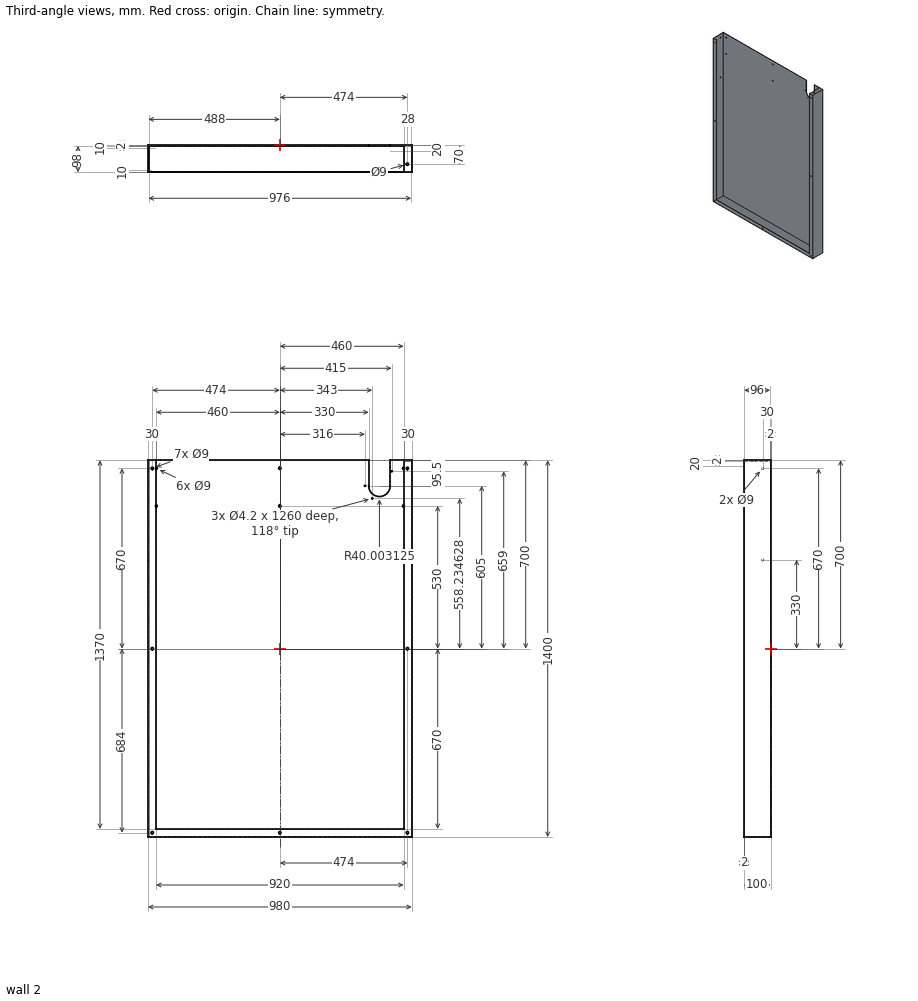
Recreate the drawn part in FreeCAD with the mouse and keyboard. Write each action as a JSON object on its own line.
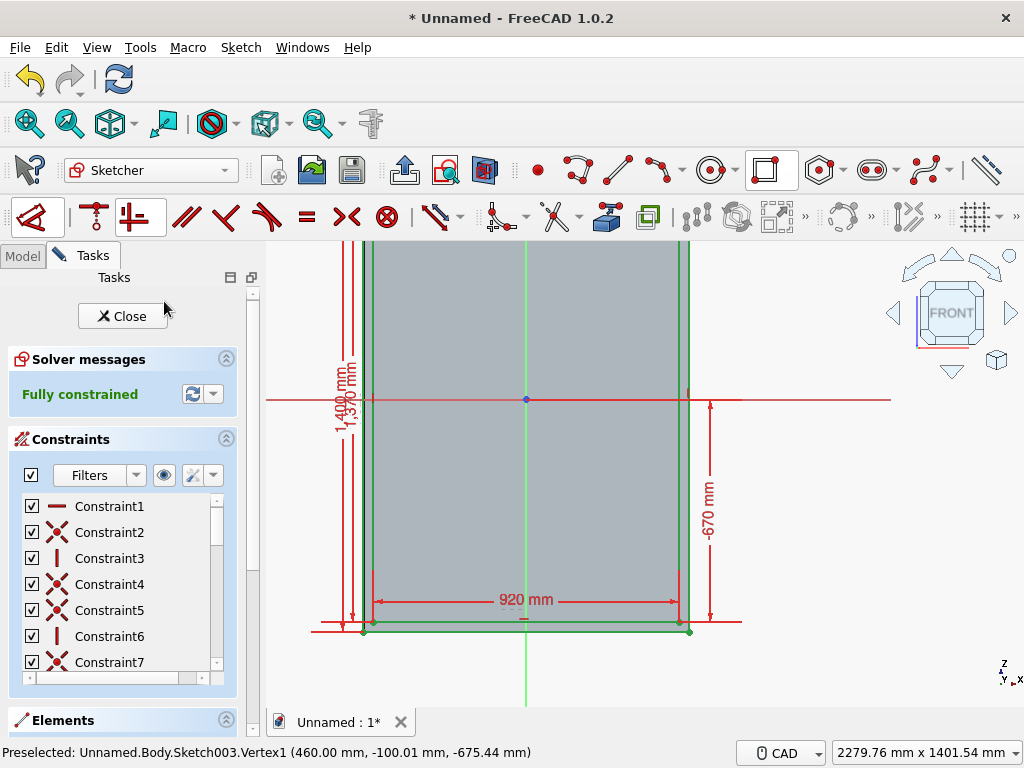
{"action": "left_click", "coordinate": [123, 316]}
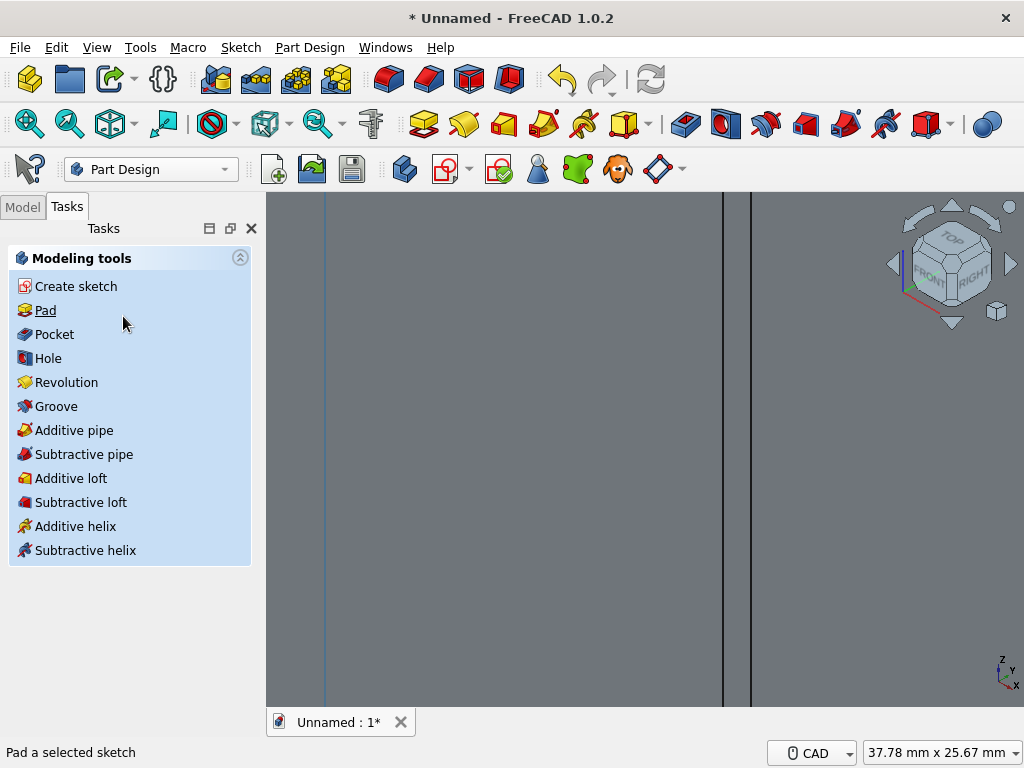
{"action": "left_click", "coordinate": [424, 124]}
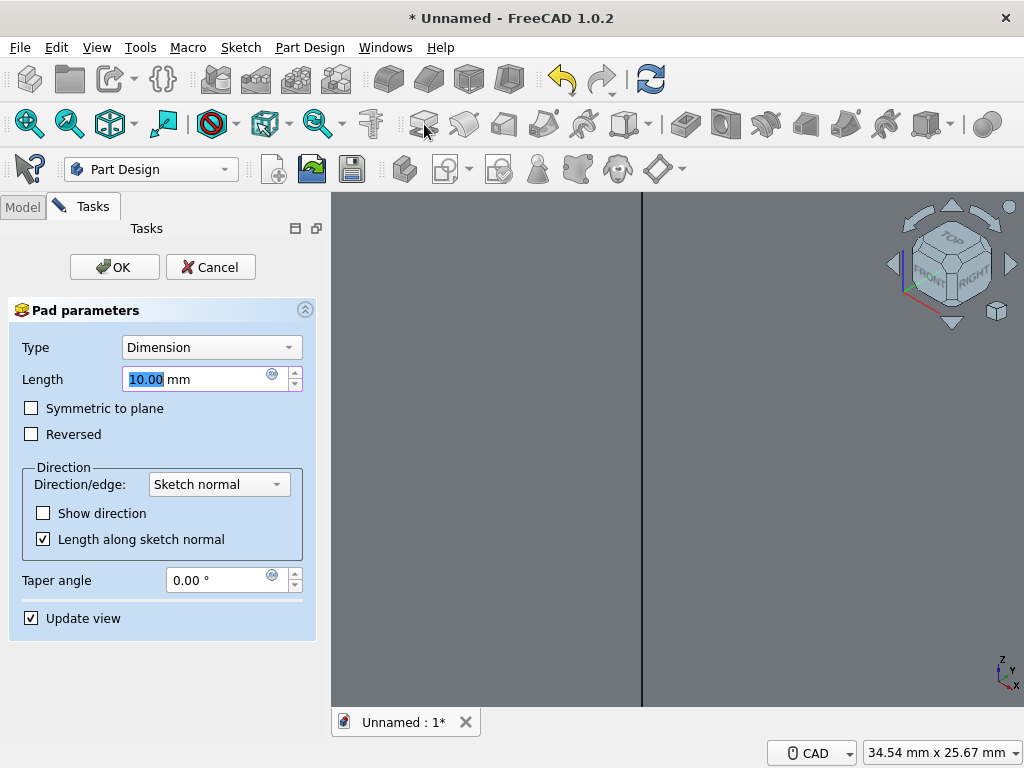
{"action": "type", "text": "2"}
{"action": "key", "text": "Tab"}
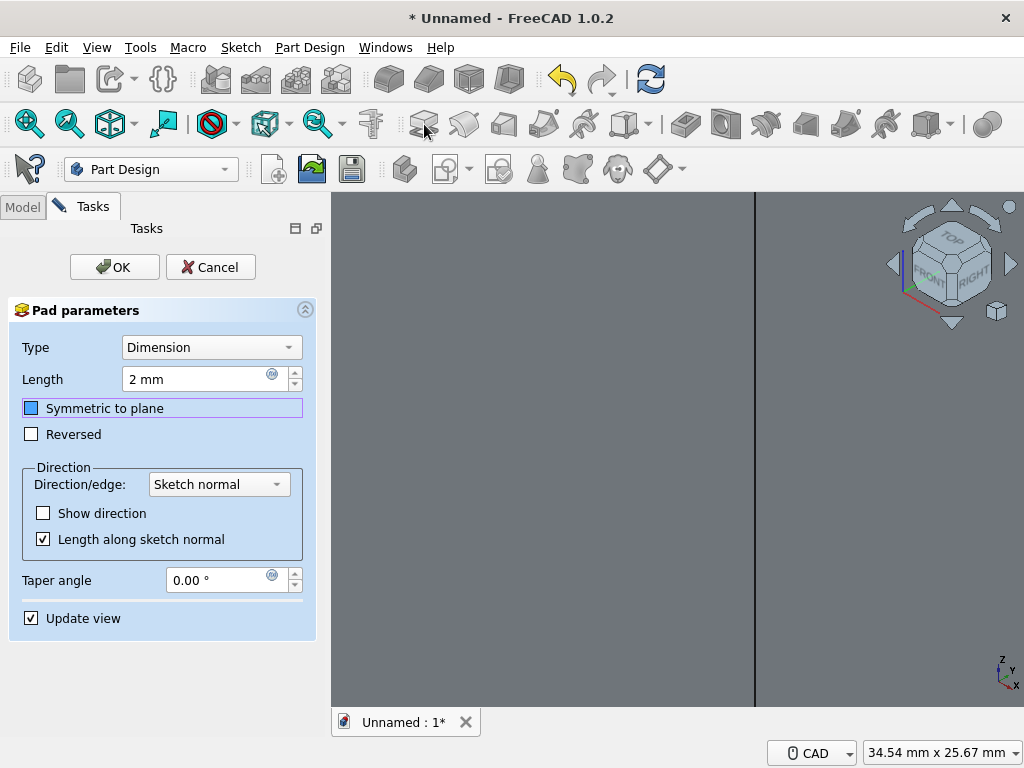
{"action": "left_click", "coordinate": [30, 434]}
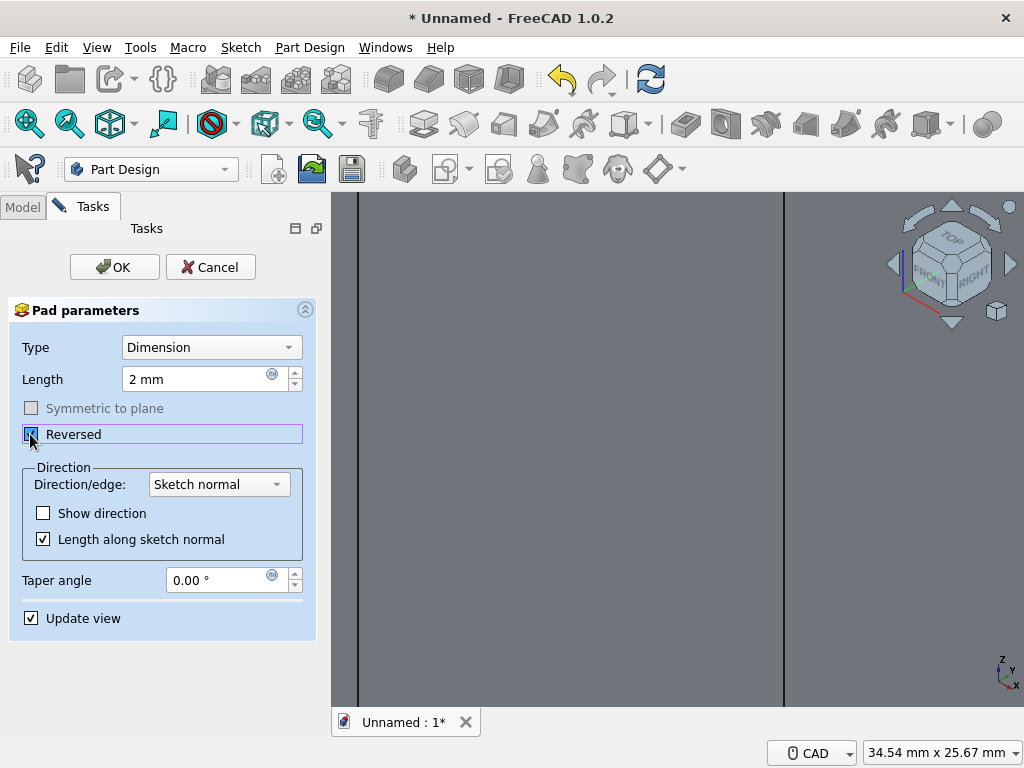
{"action": "left_click", "coordinate": [115, 267]}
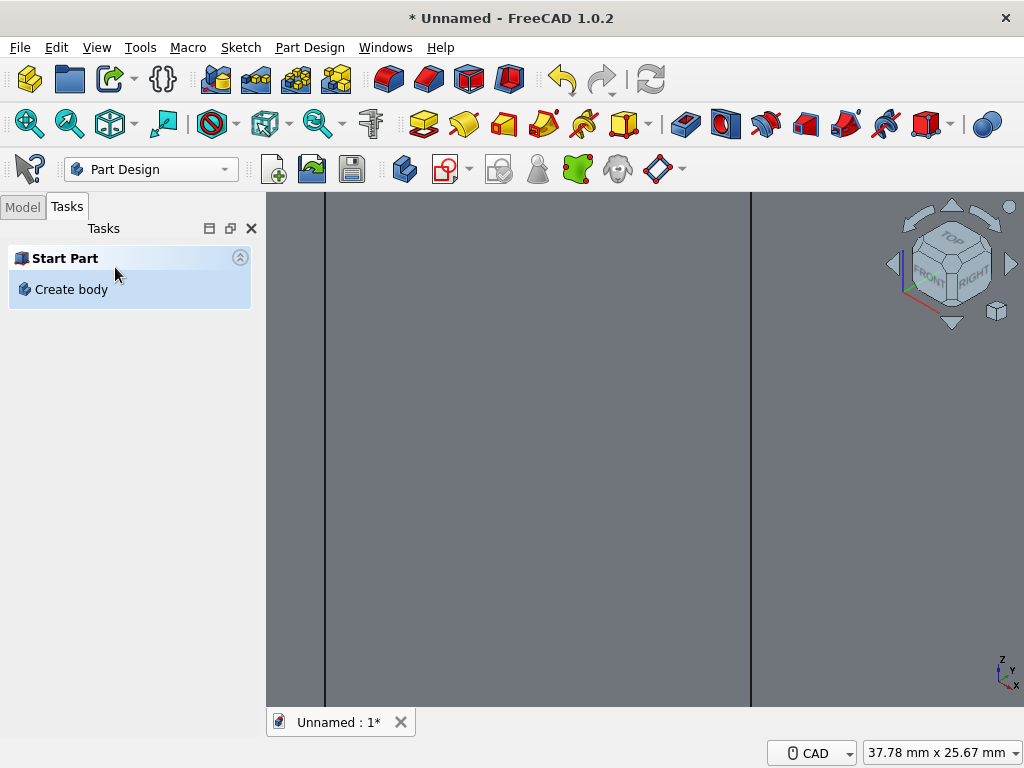
{"action": "left_click", "coordinate": [30, 124]}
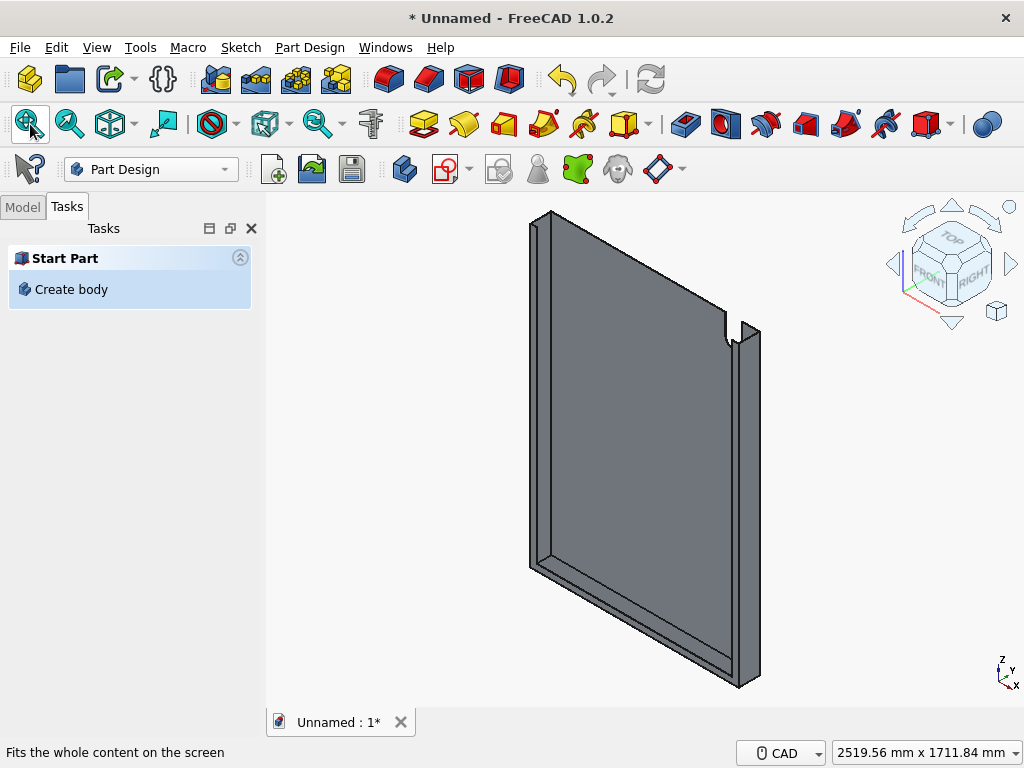
{"action": "left_click", "coordinate": [23, 206]}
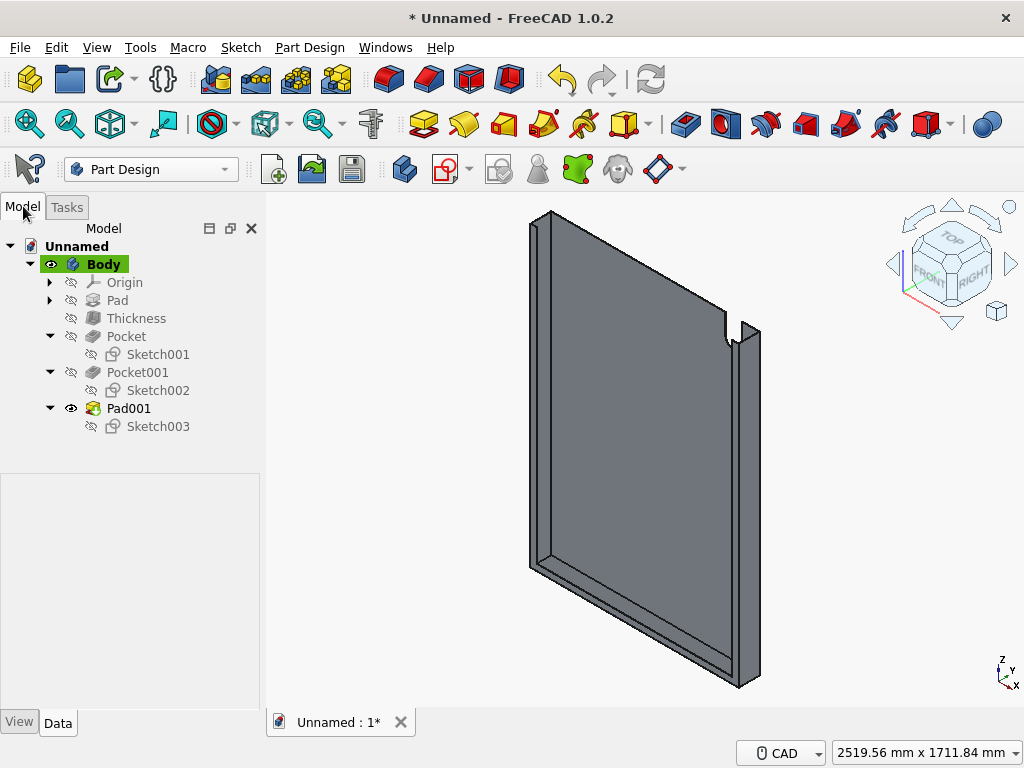
{"action": "left_click", "coordinate": [50, 282]}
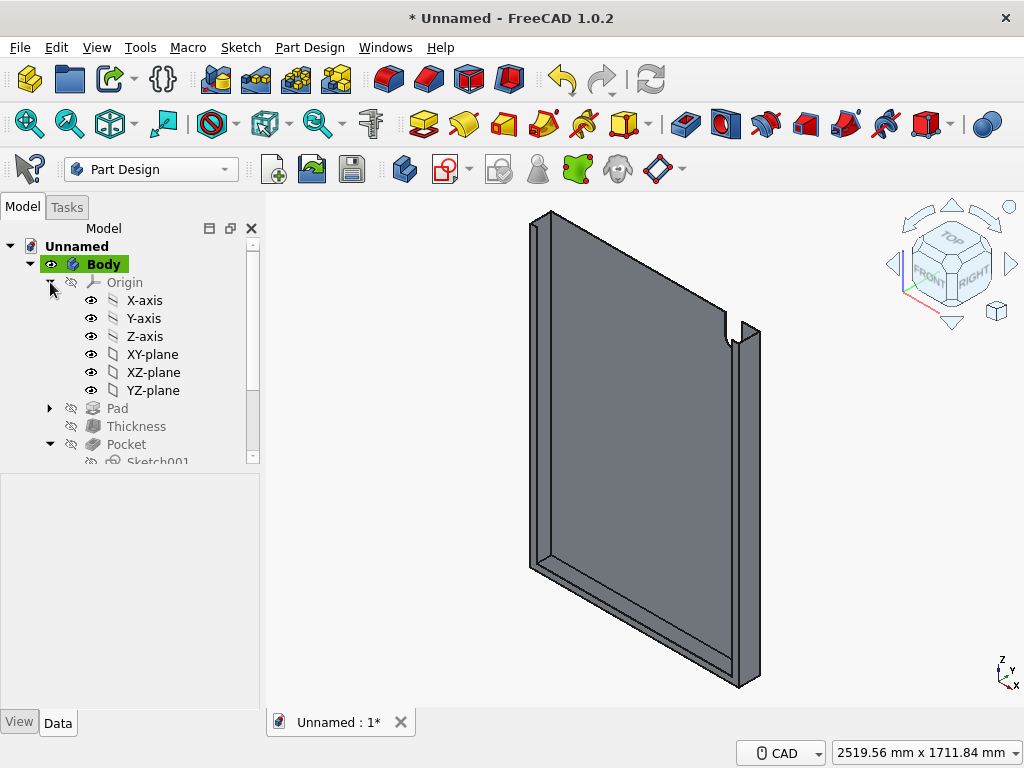
{"action": "left_click", "coordinate": [136, 390]}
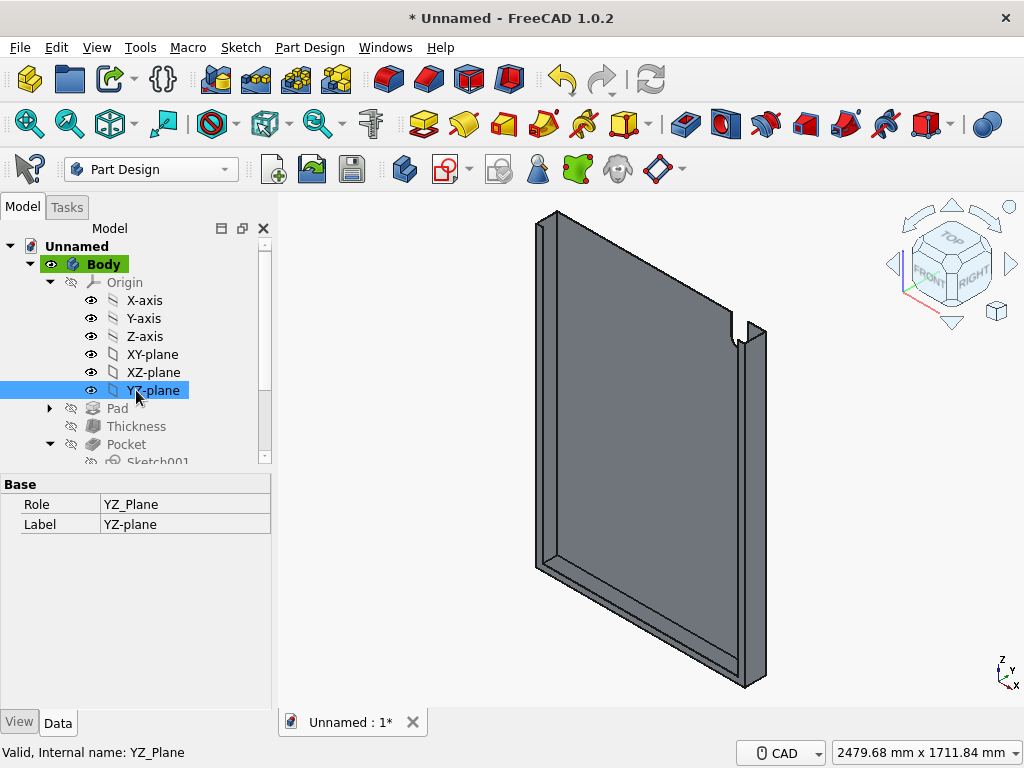
{"action": "left_click", "coordinate": [658, 170]}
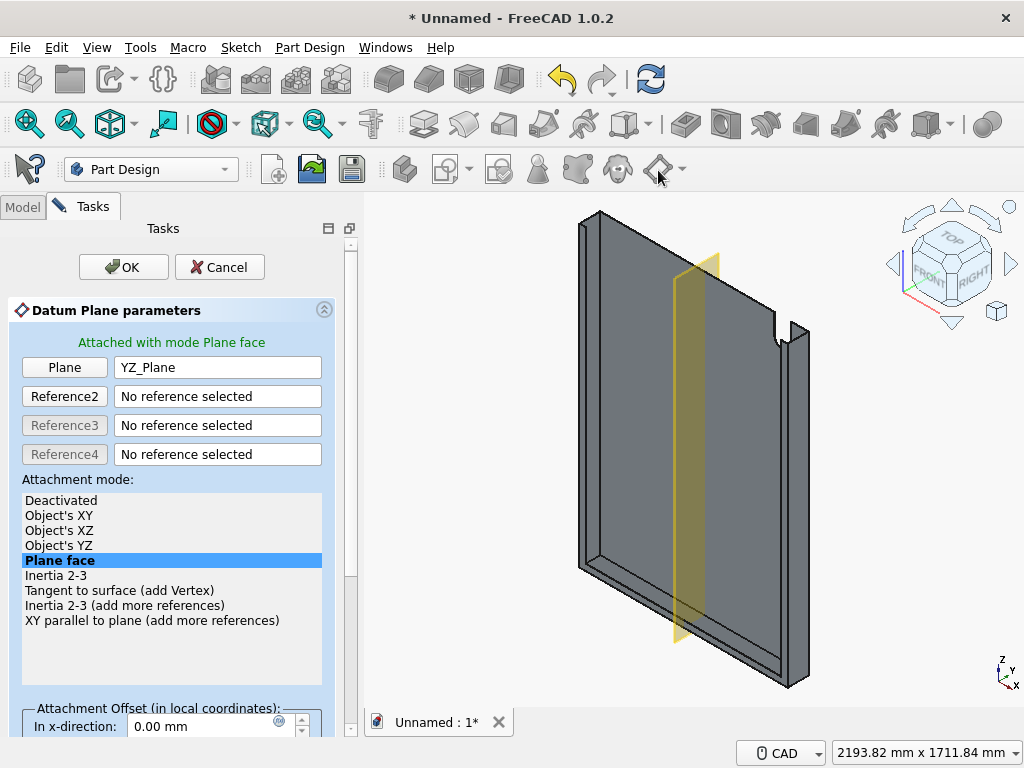
{"action": "scroll", "coordinate": [351, 487], "scroll_direction": "down", "scroll_amount": 3}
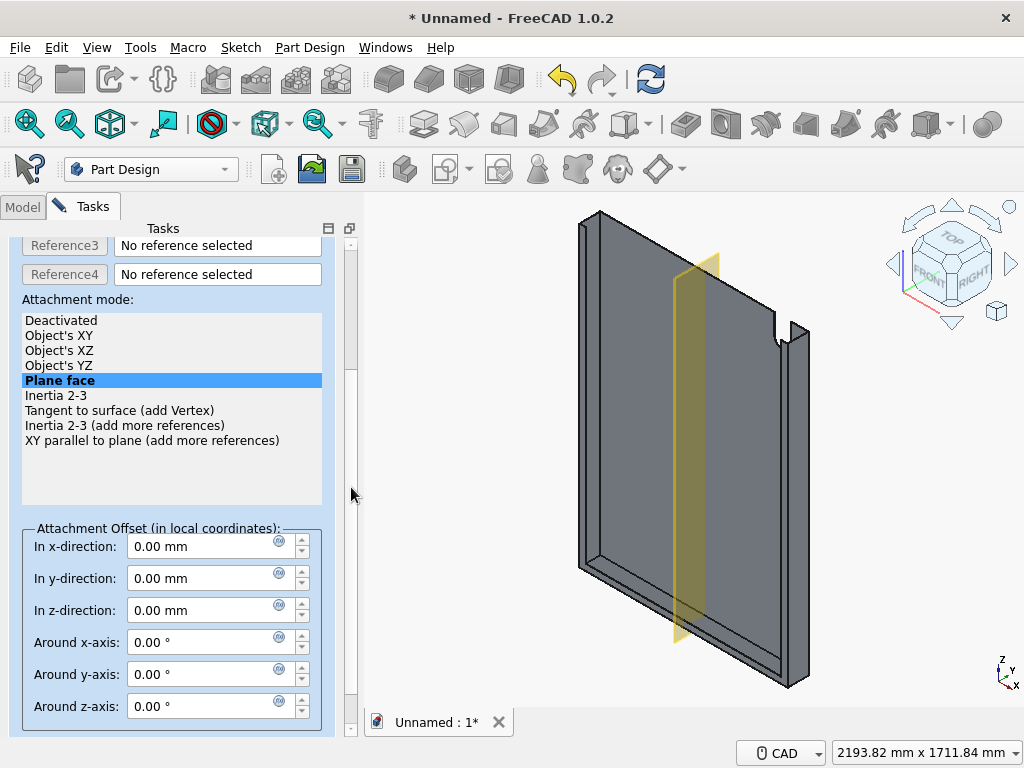
{"action": "triple_click", "coordinate": [210, 610]}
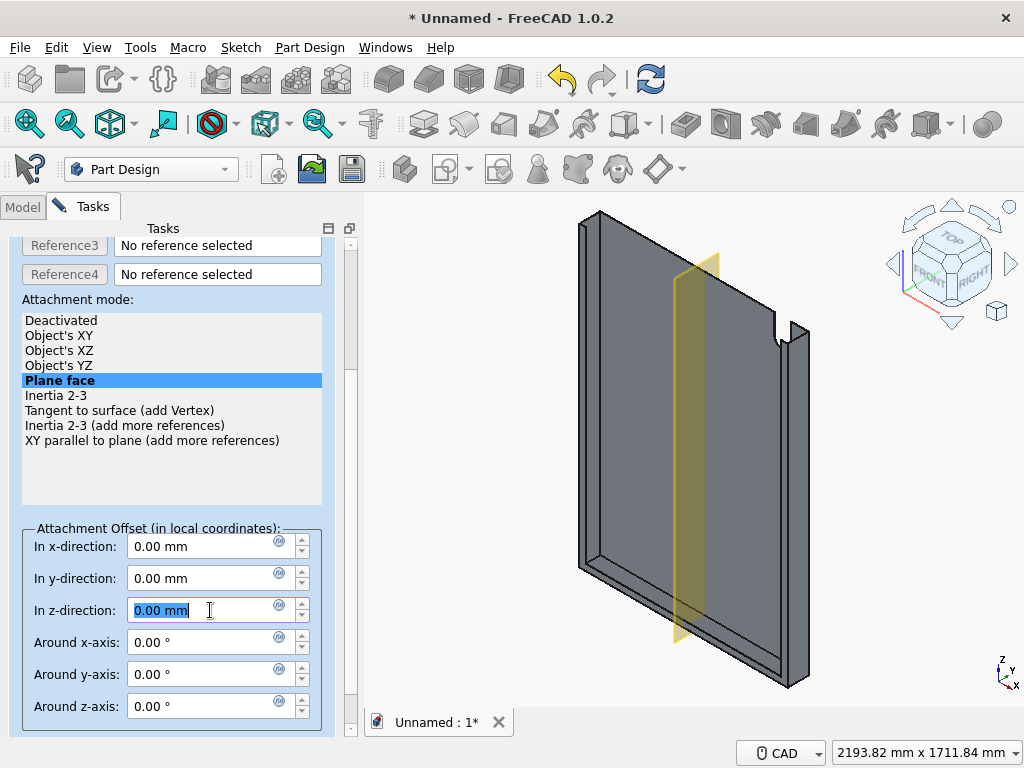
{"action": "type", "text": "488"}
{"action": "key", "text": "Tab"}